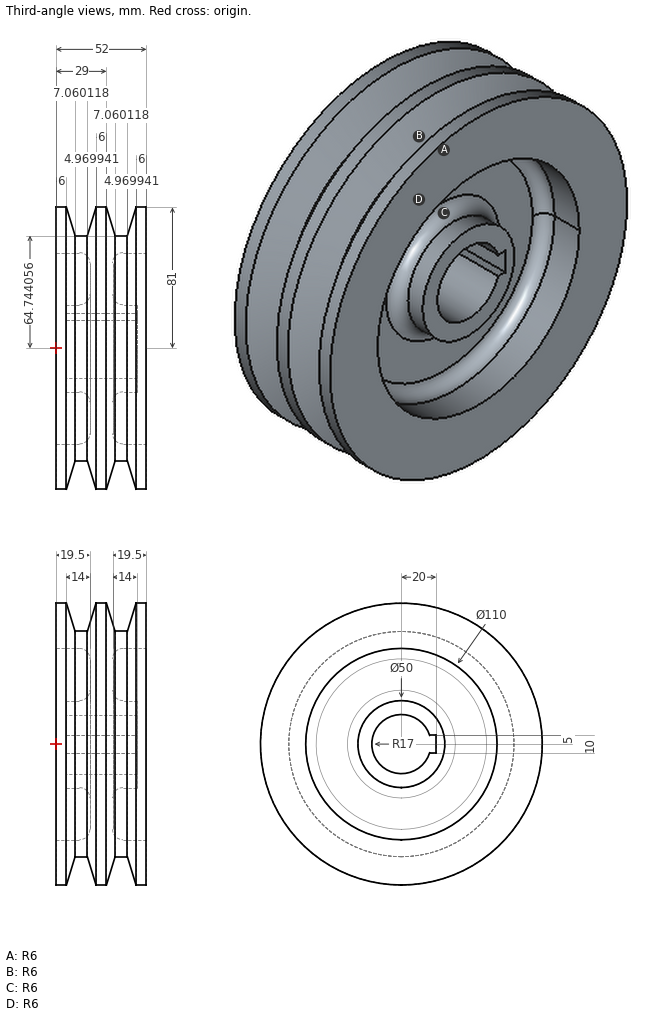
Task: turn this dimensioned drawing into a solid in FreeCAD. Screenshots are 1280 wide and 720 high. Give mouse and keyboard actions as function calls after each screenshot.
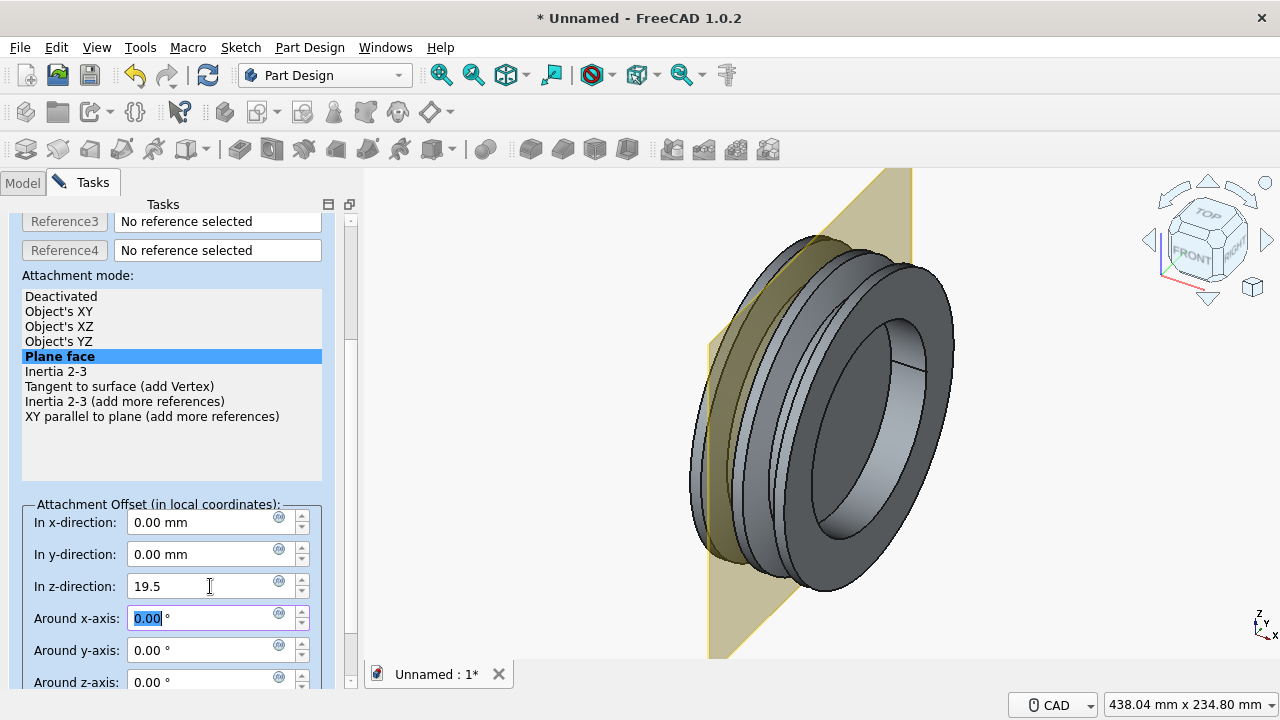
scroll(351, 451, up, 4)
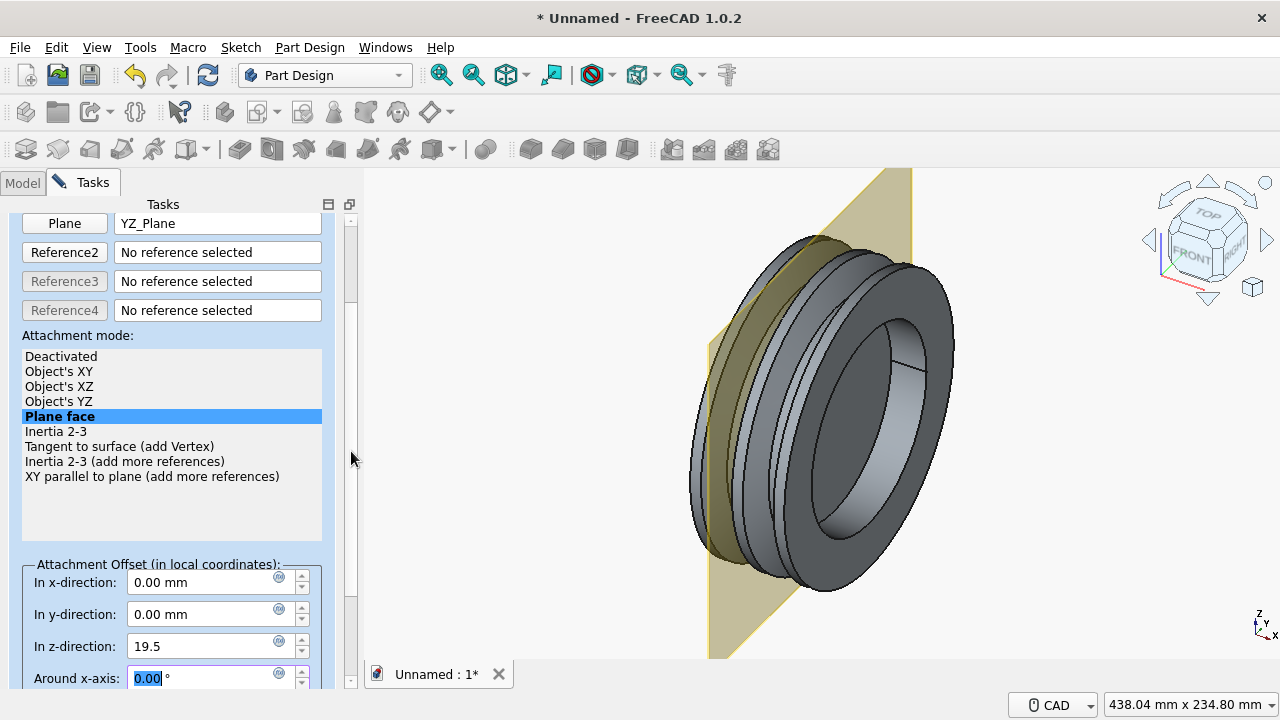
click(124, 243)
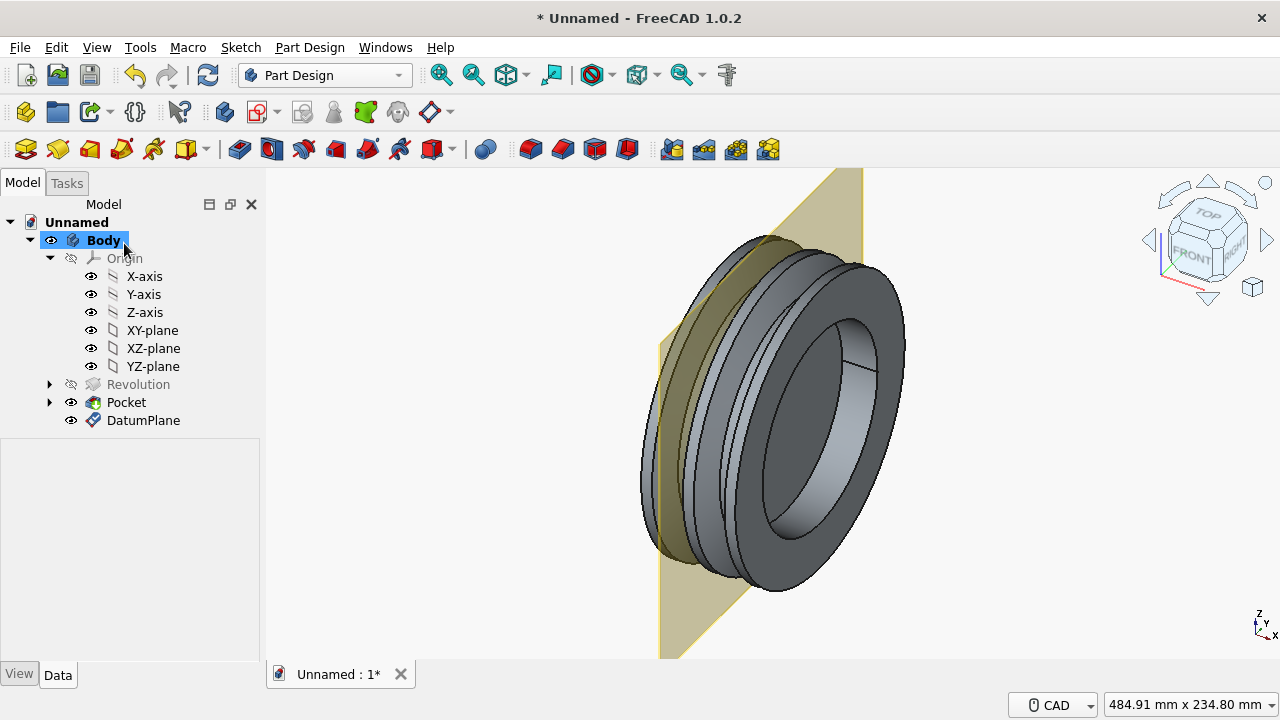
click(116, 420)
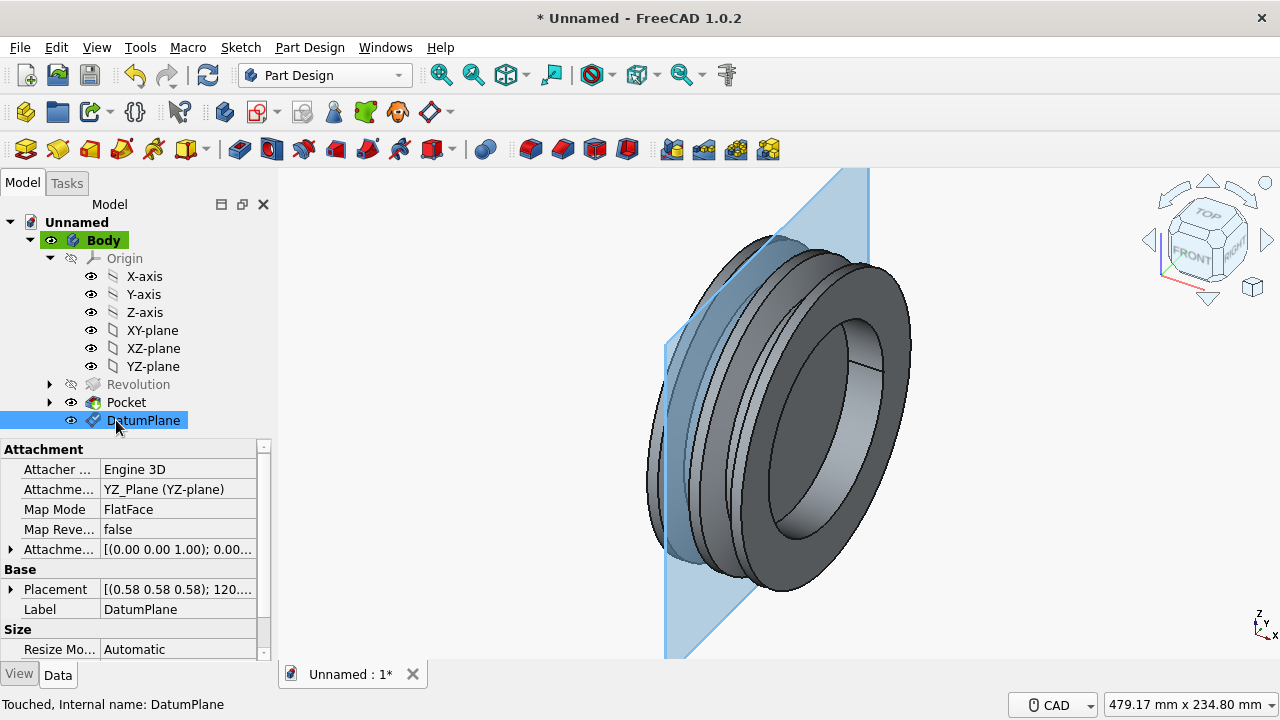
click(258, 112)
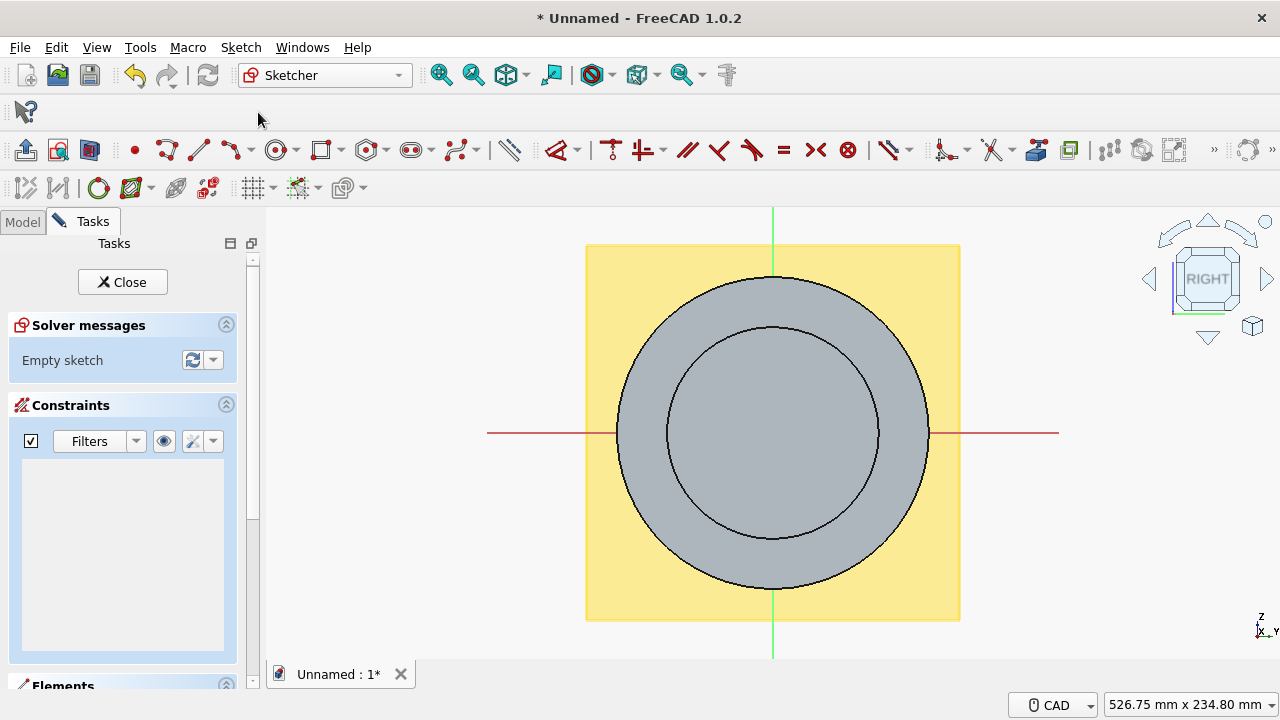
key(q)
key(s)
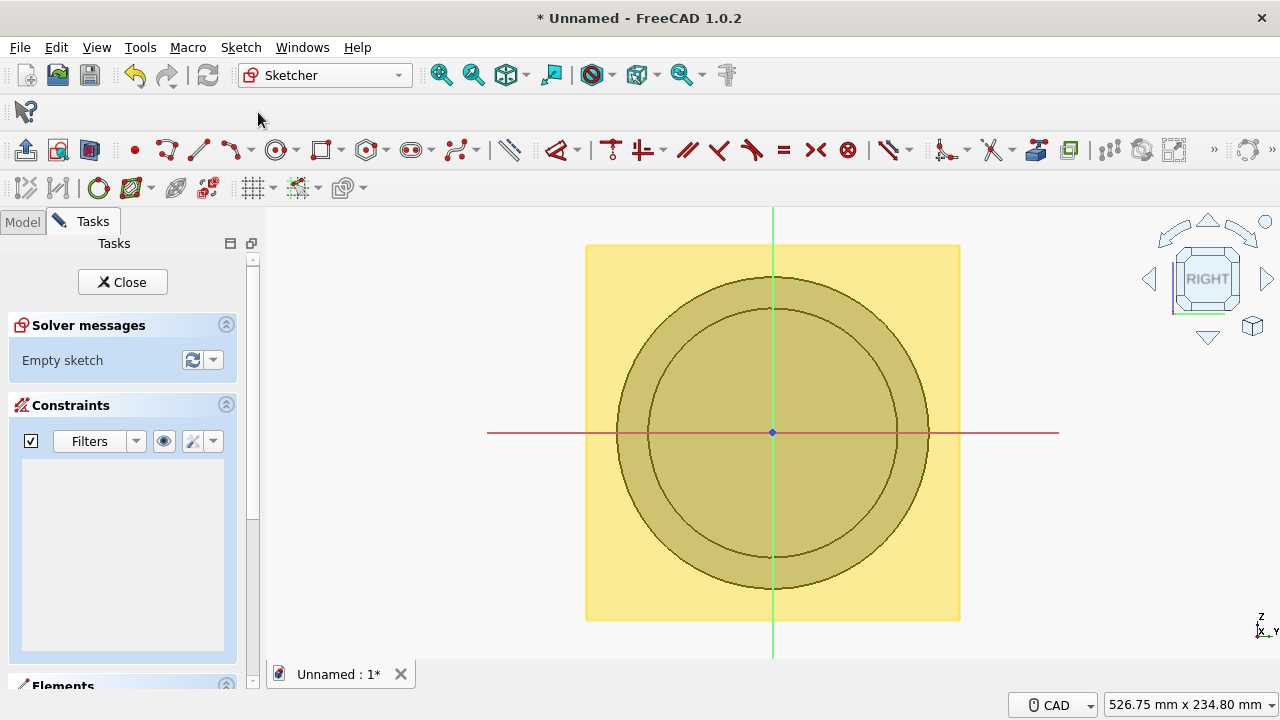
key(g)
key(c)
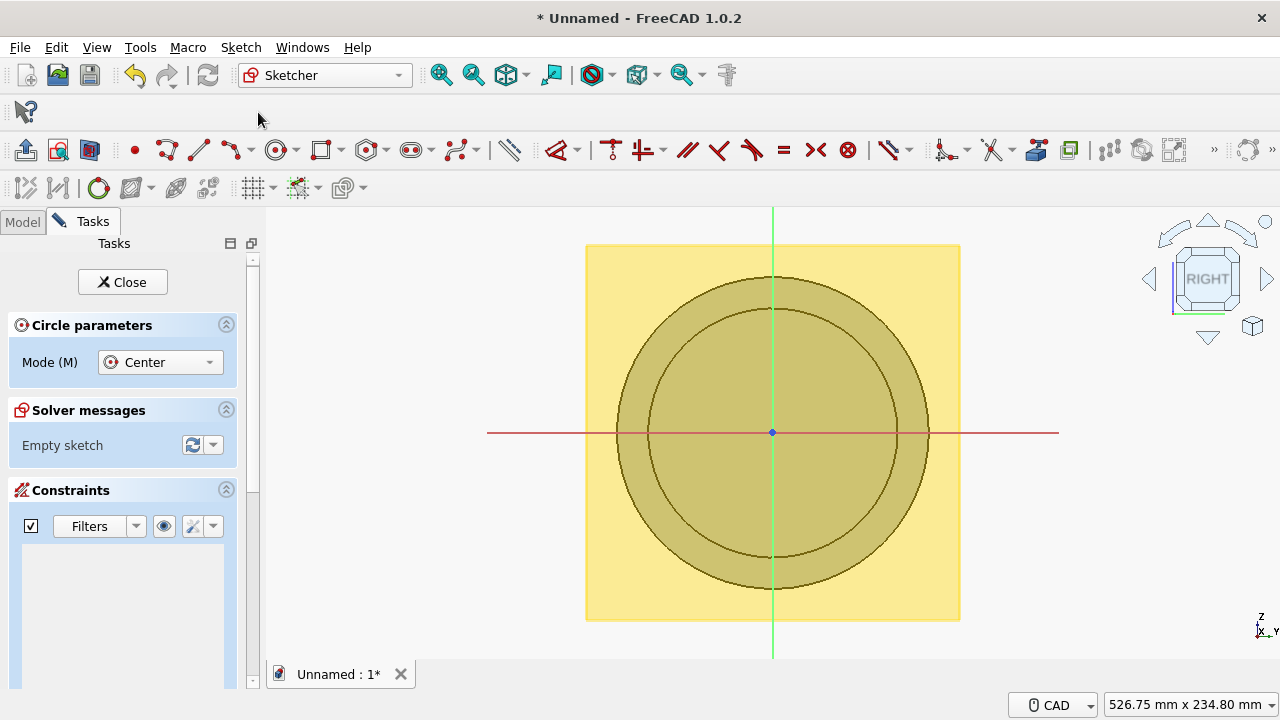
click(773, 433)
click(848, 358)
key(Escape)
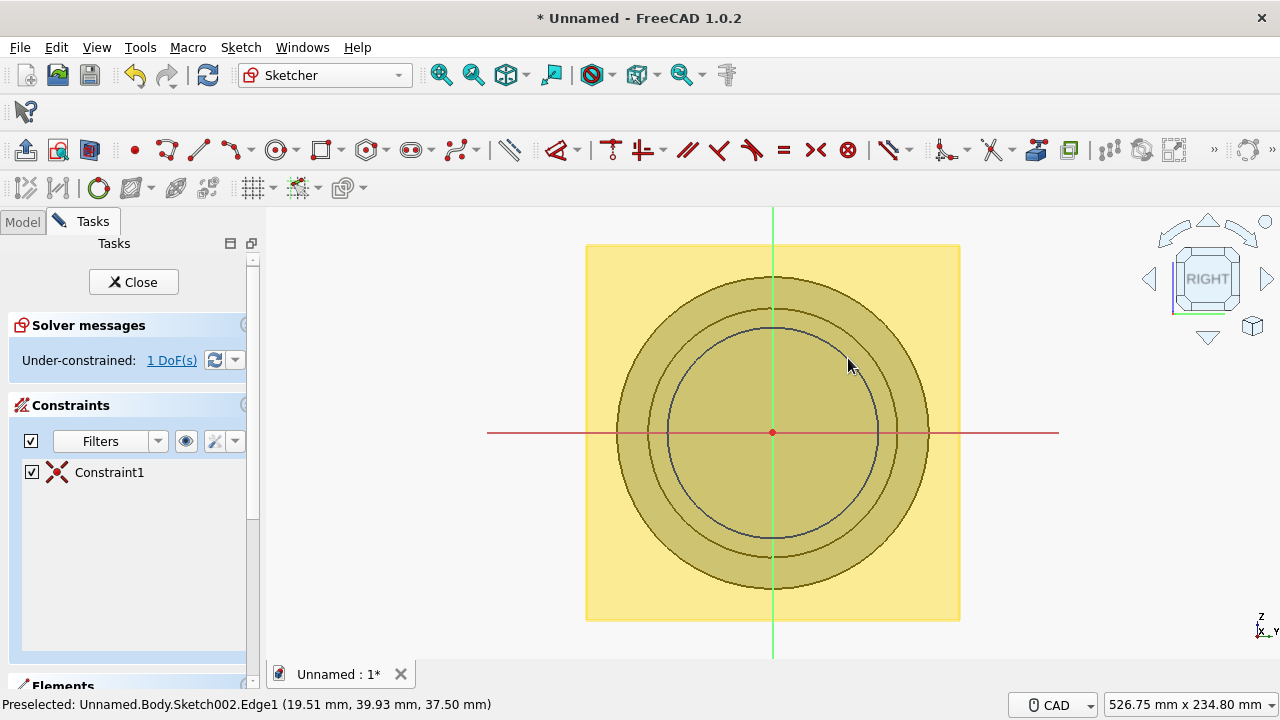
key(d)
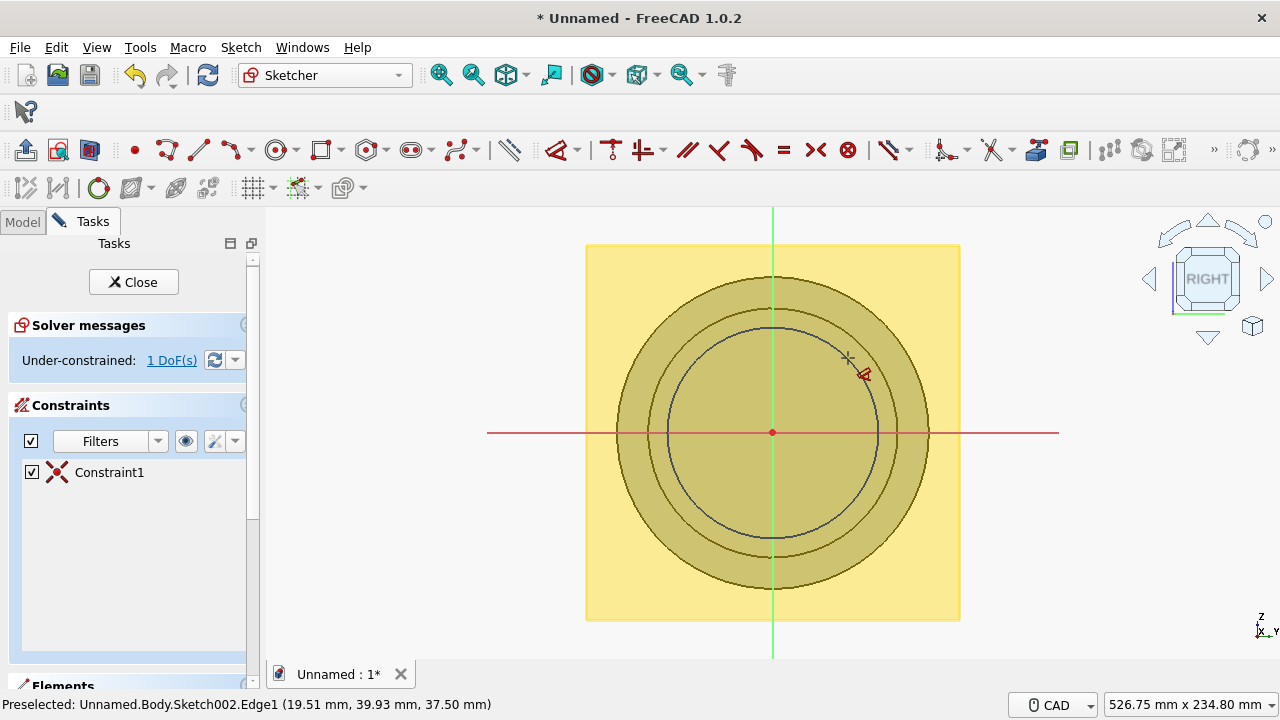
click(847, 358)
click(869, 335)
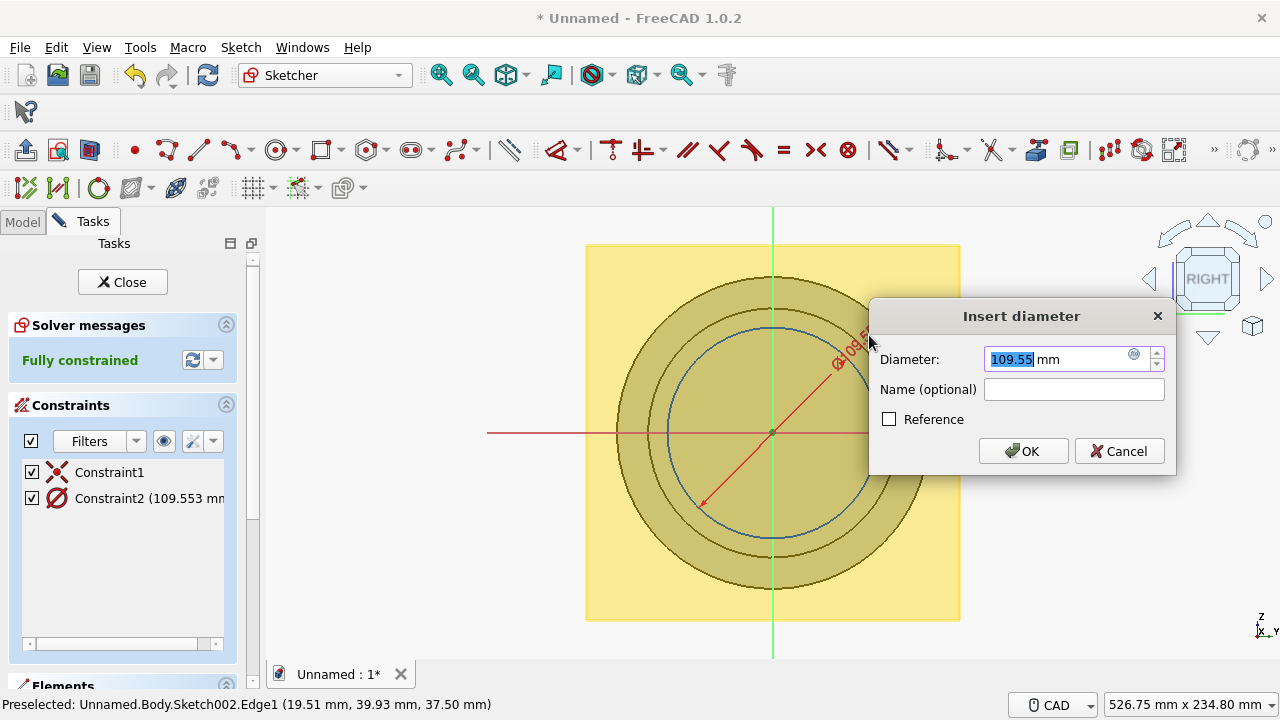
text(110)
key(Return)
key(Escape)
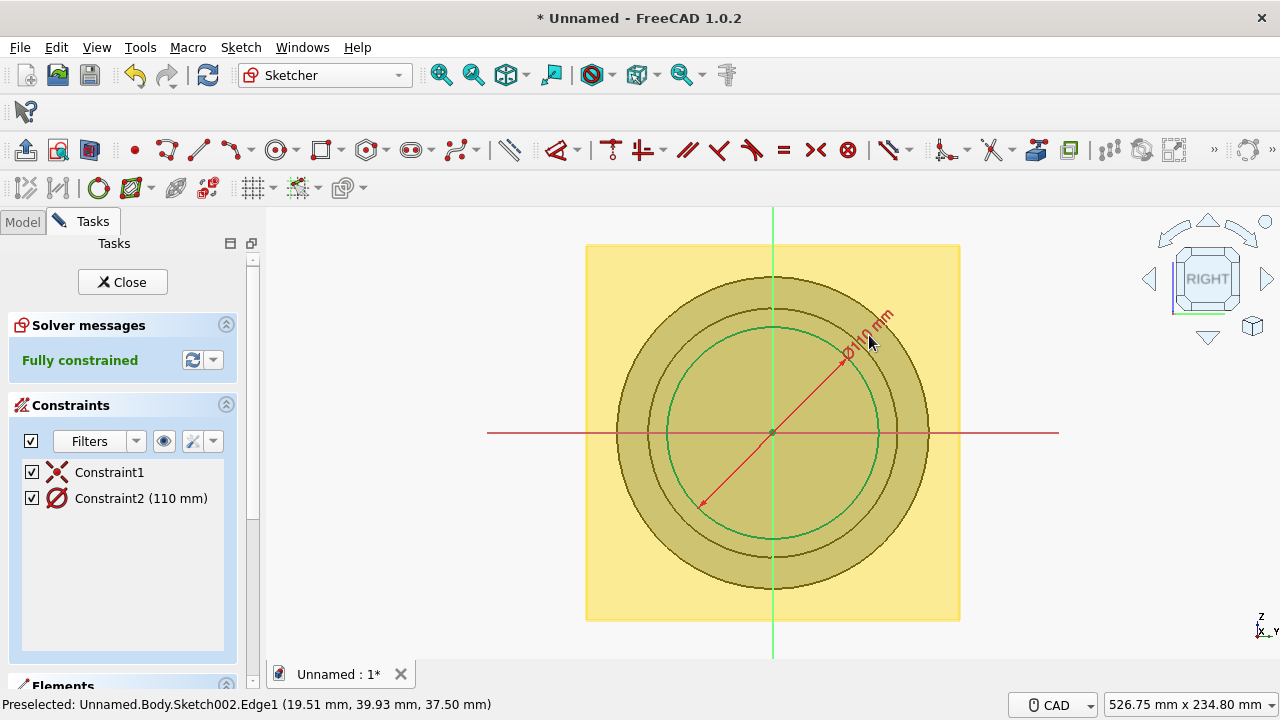
click(123, 282)